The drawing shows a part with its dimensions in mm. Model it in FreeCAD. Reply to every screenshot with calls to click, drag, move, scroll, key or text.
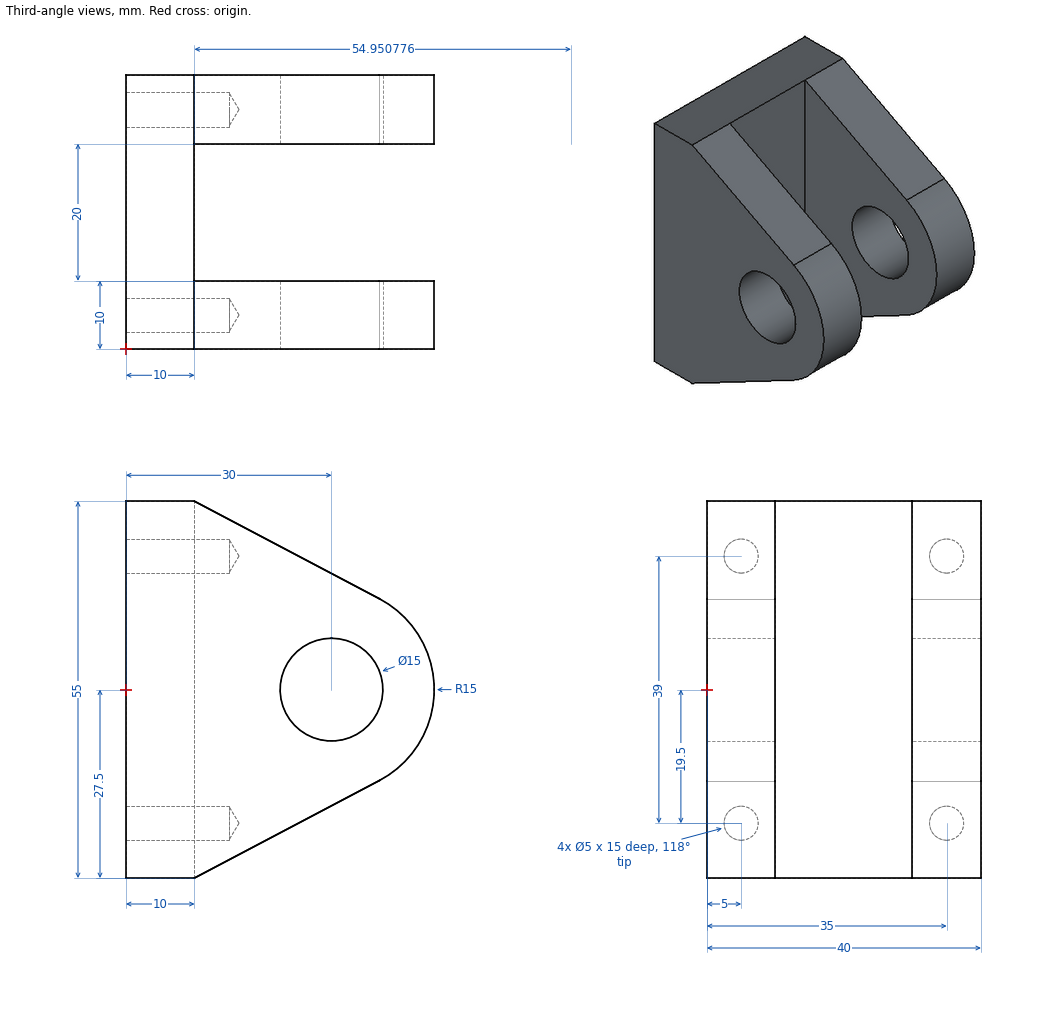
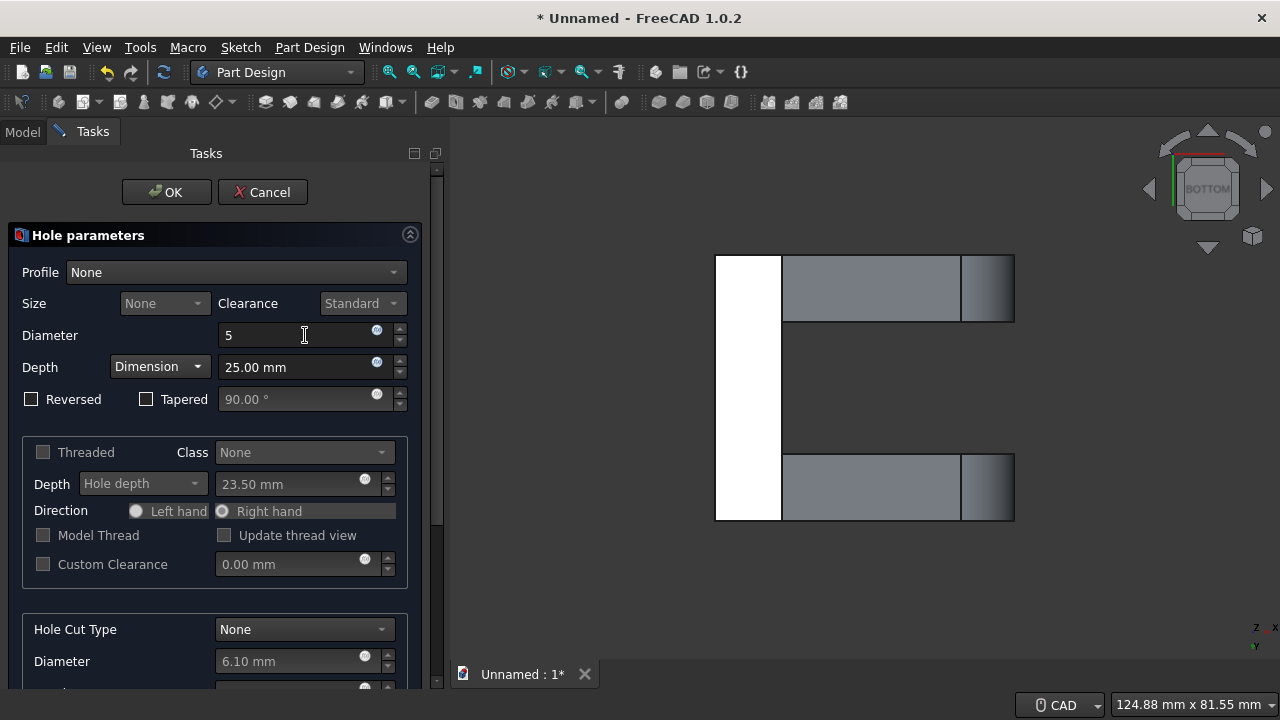
triple_click(305, 367)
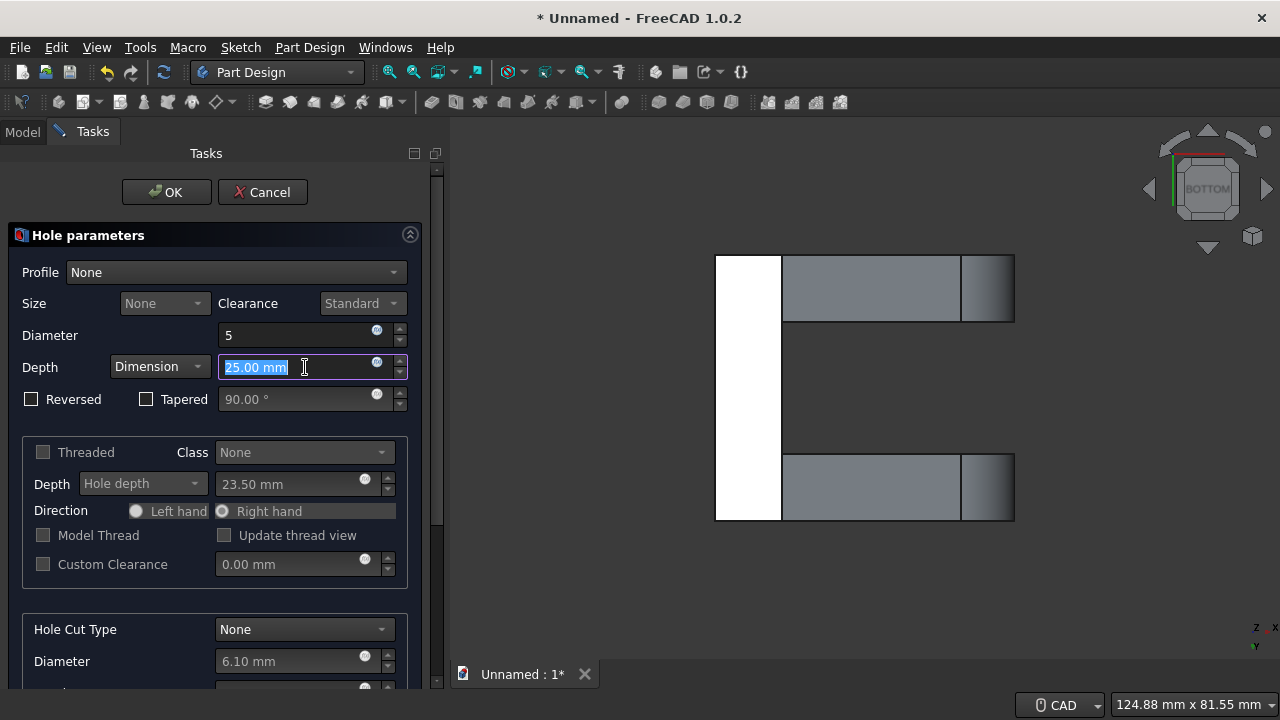
text(15)
key(Tab)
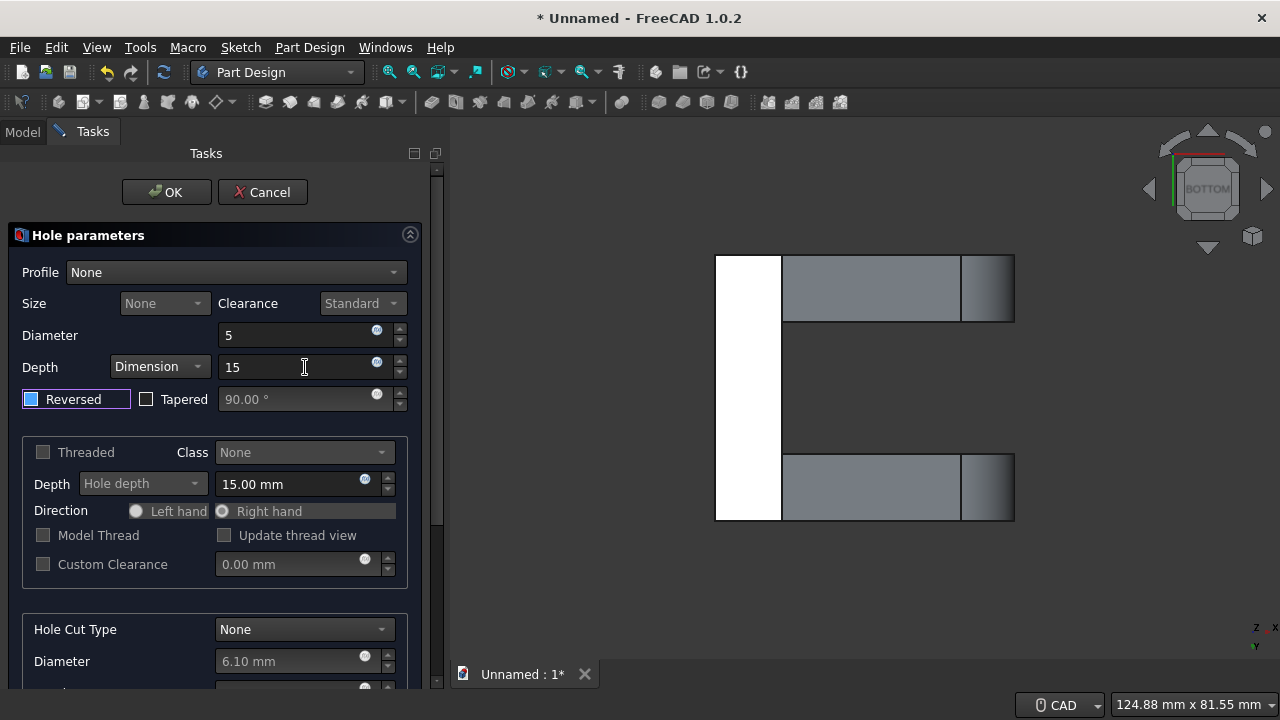
click(30, 399)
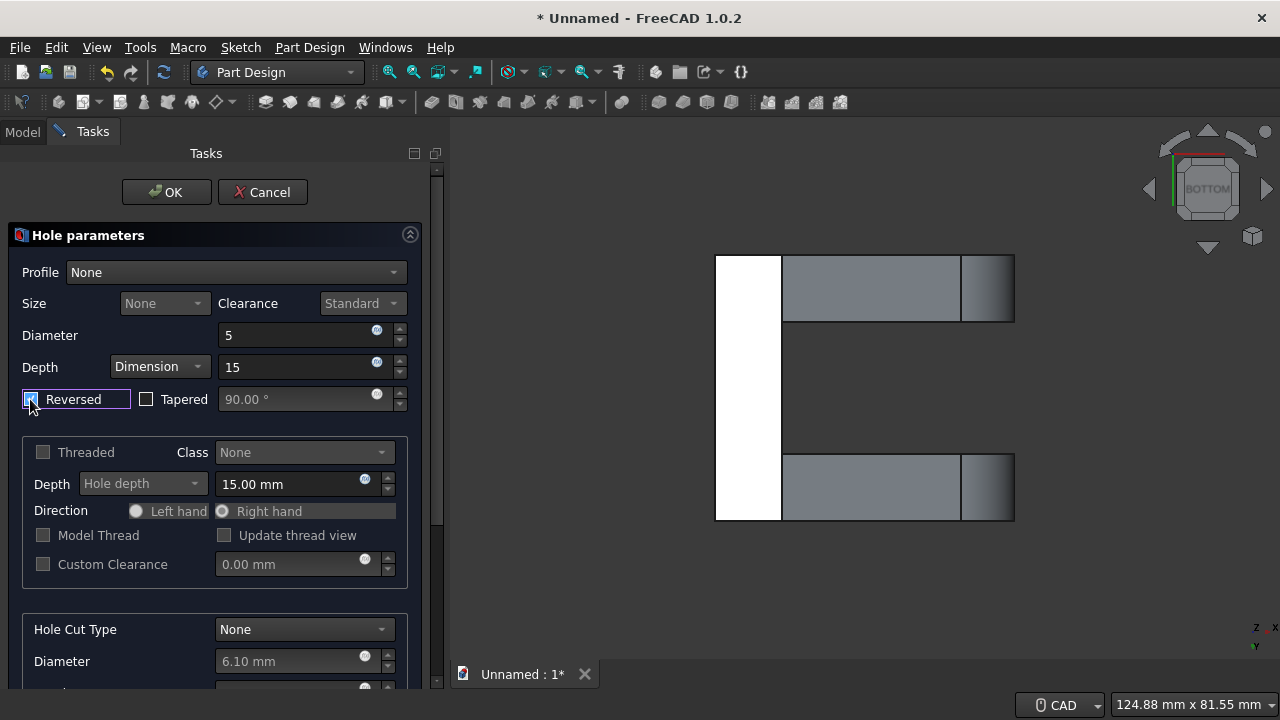
click(167, 192)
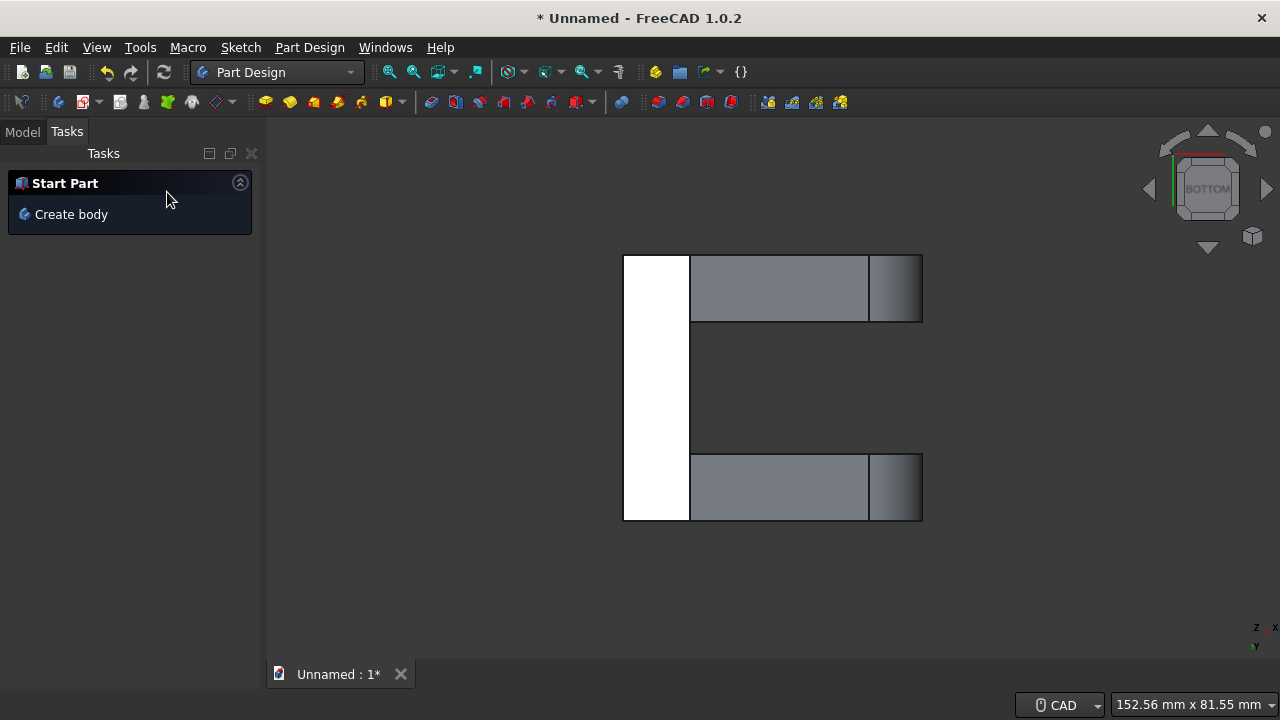
key(0)